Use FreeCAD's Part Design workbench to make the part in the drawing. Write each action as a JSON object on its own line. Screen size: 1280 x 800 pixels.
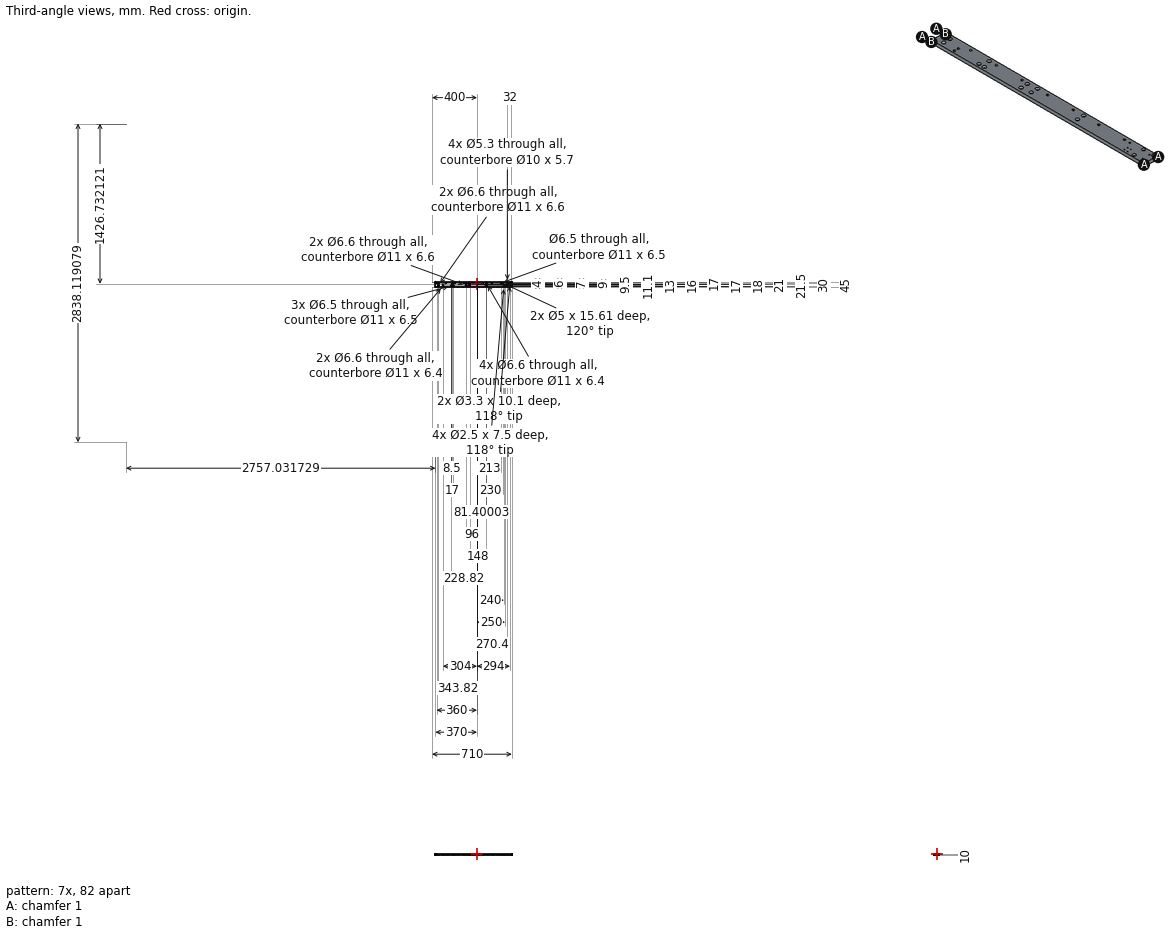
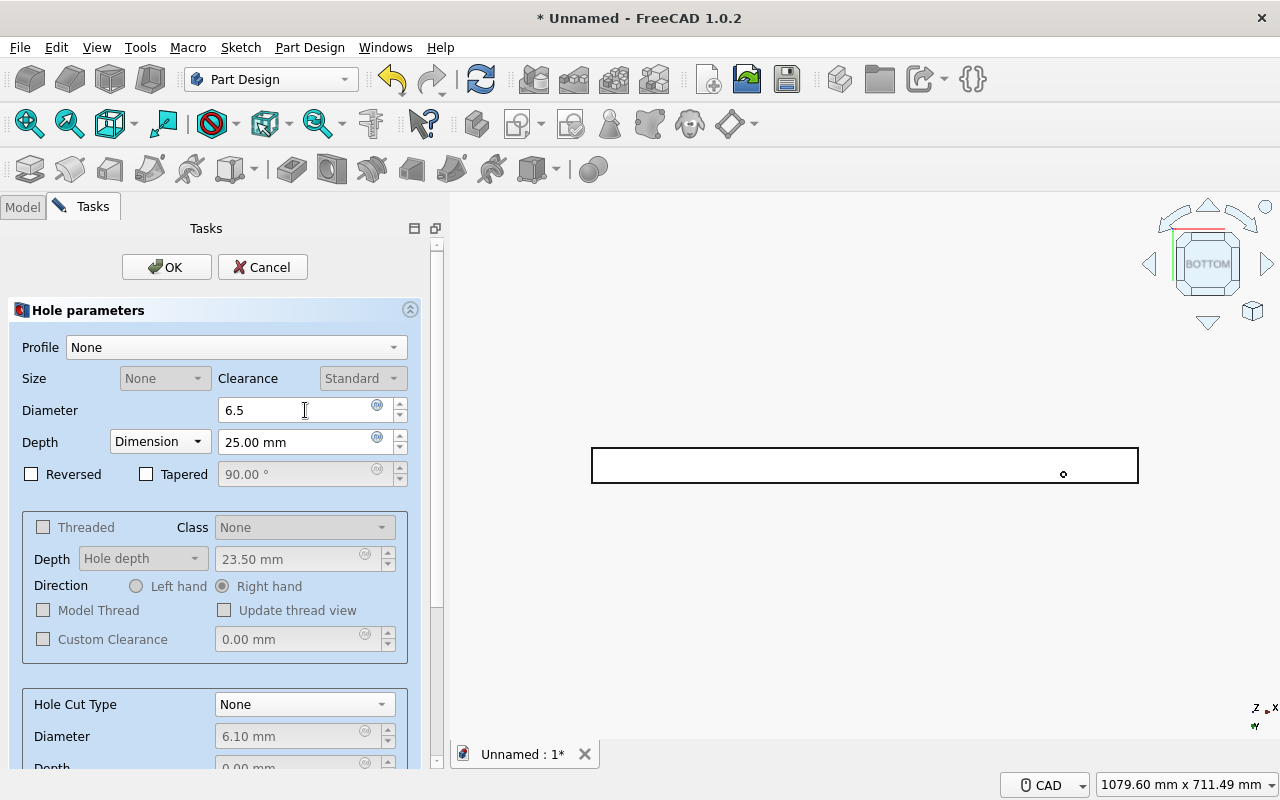
{"action": "left_click", "coordinate": [161, 442]}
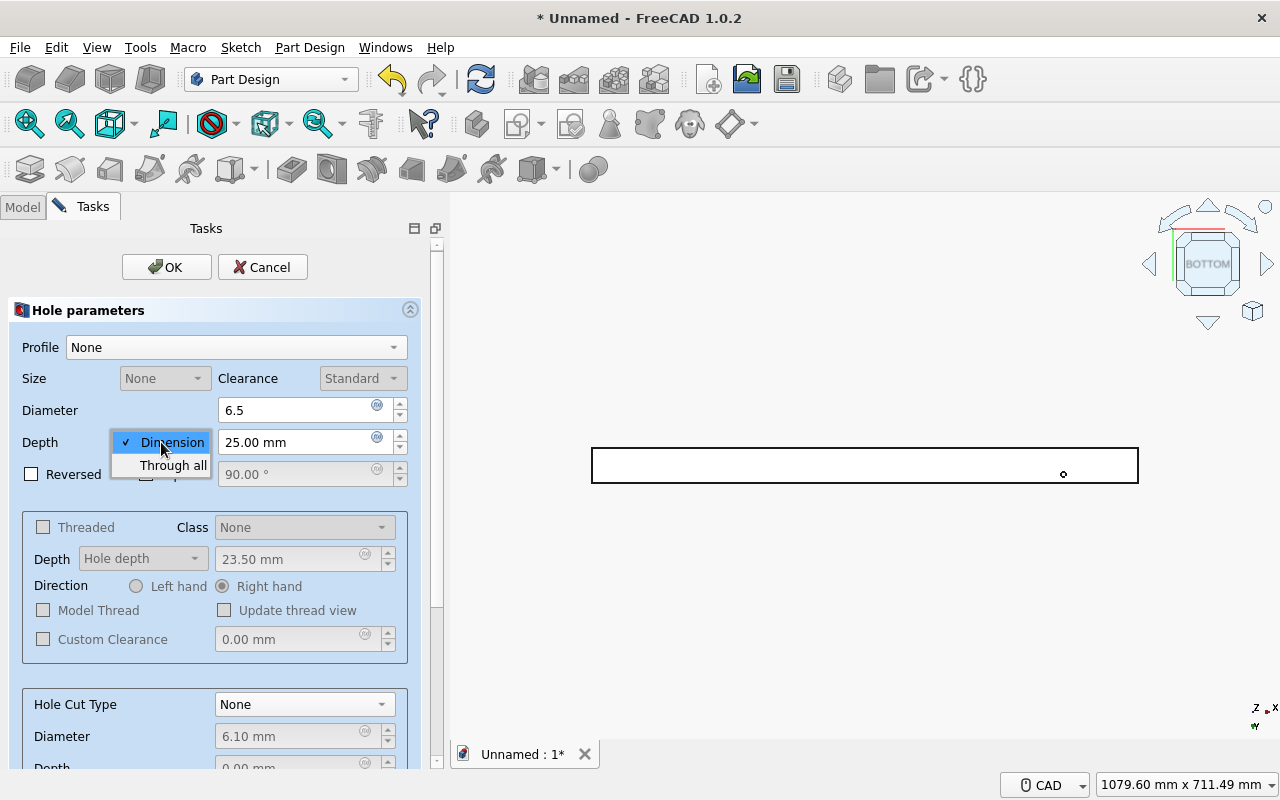
{"action": "left_click", "coordinate": [160, 466]}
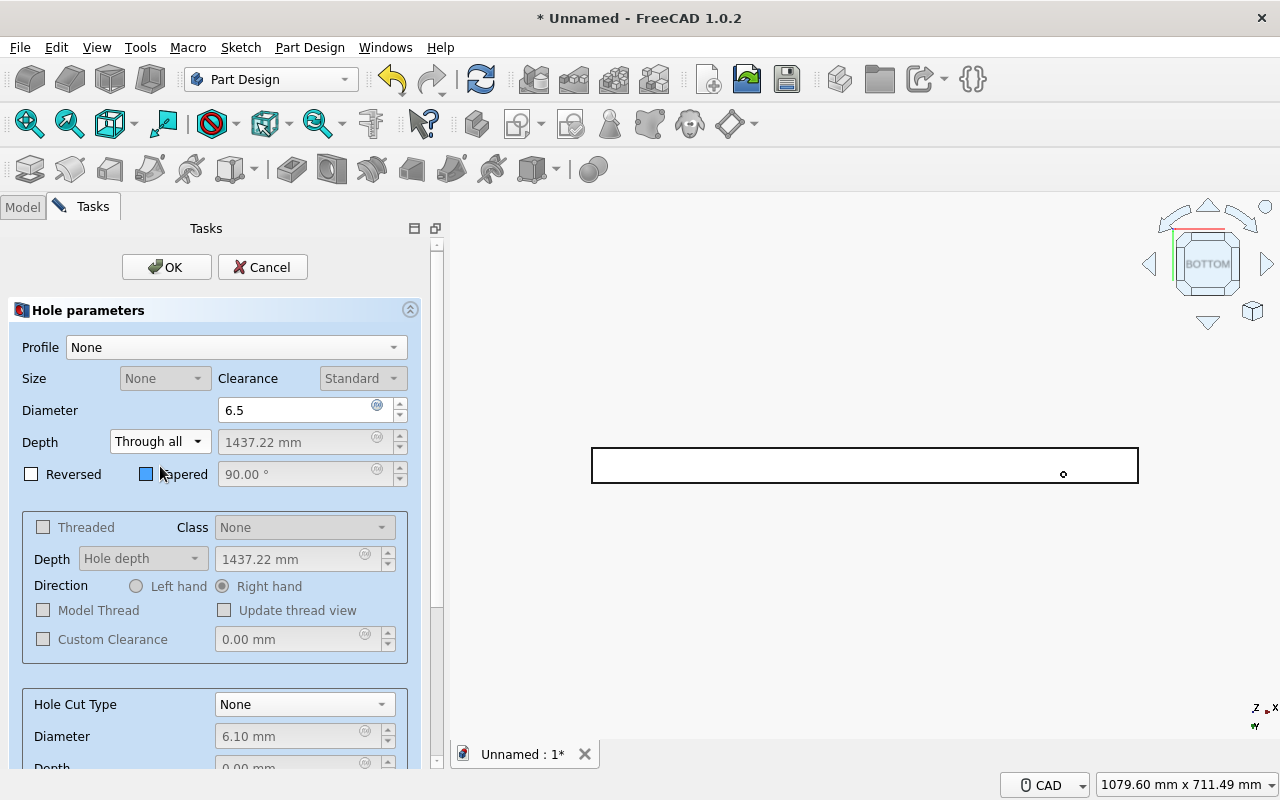
{"action": "left_click", "coordinate": [306, 704]}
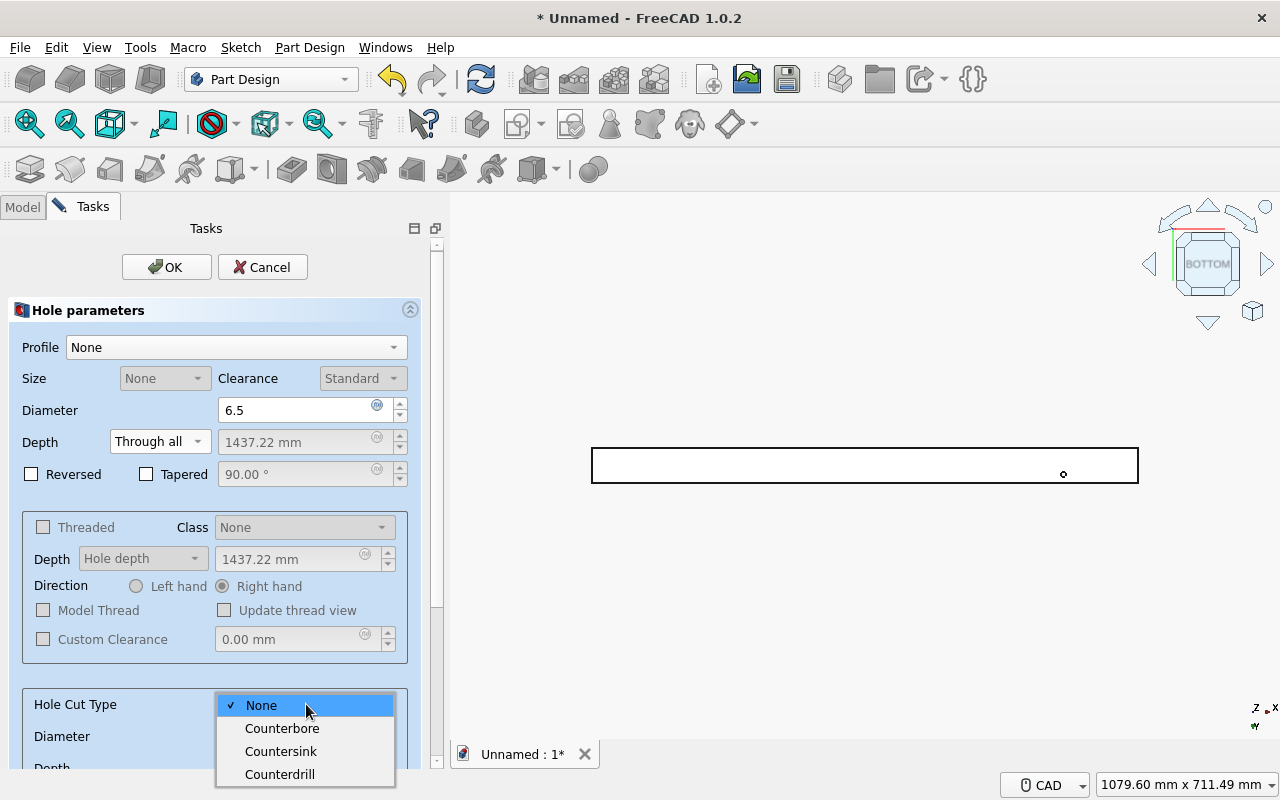
{"action": "left_click", "coordinate": [304, 728]}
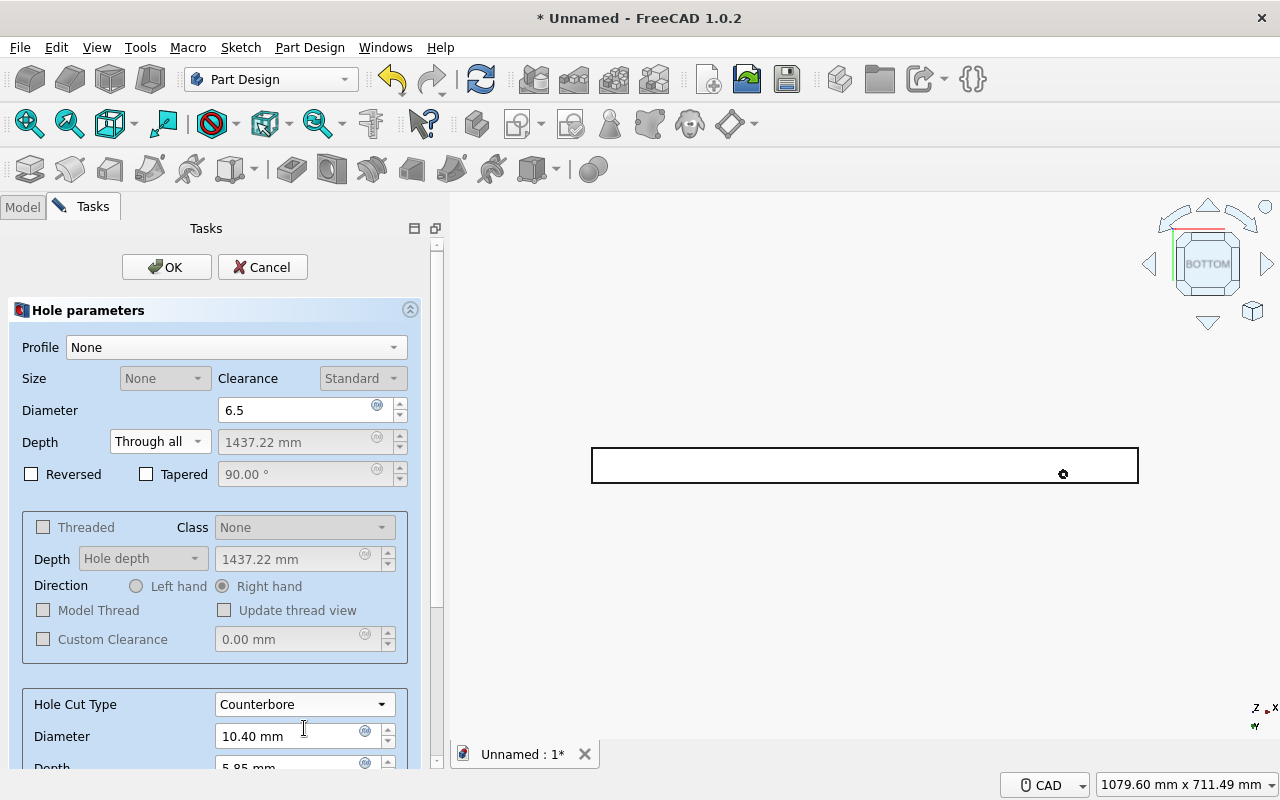
{"action": "triple_click", "coordinate": [298, 736]}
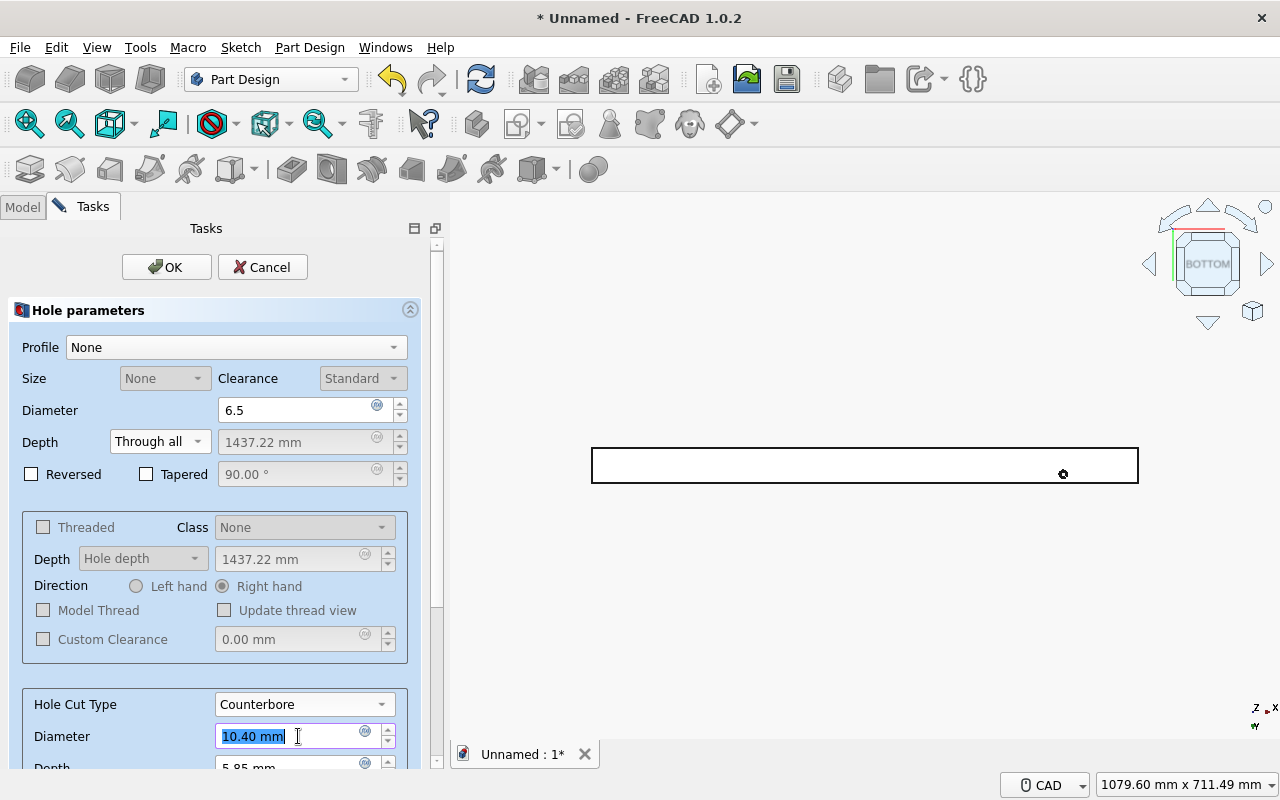
{"action": "type", "text": "11"}
{"action": "key", "text": "Tab"}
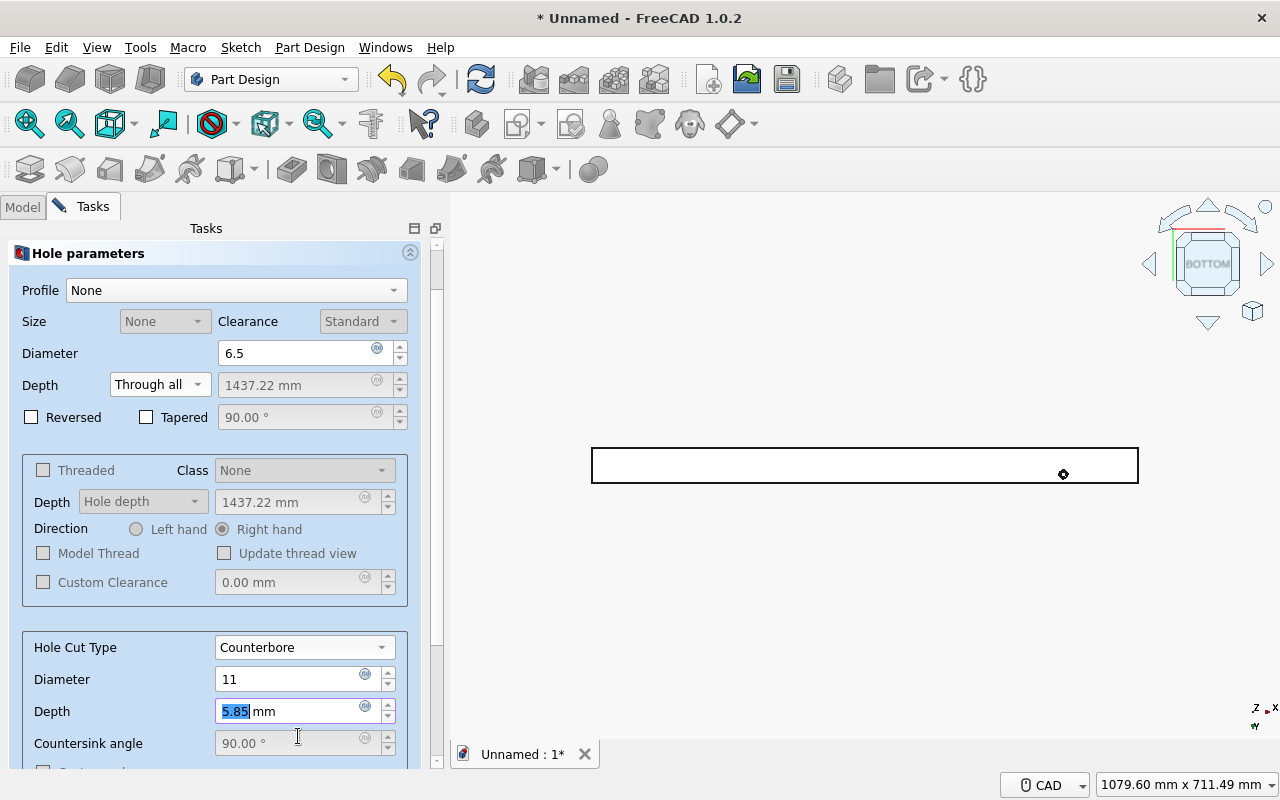
{"action": "type", "text": "6.5"}
{"action": "key", "text": "Tab"}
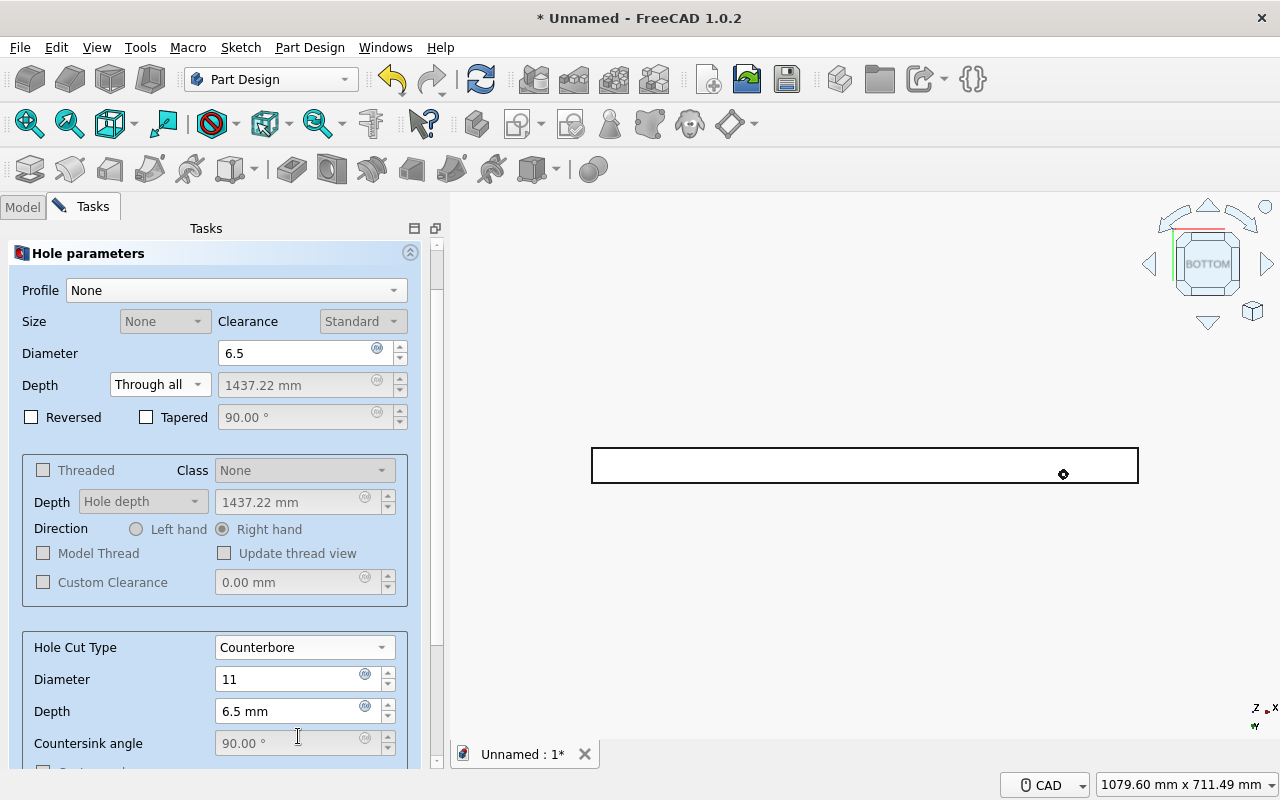
{"action": "scroll", "coordinate": [437, 503], "scroll_direction": "up", "scroll_amount": 2}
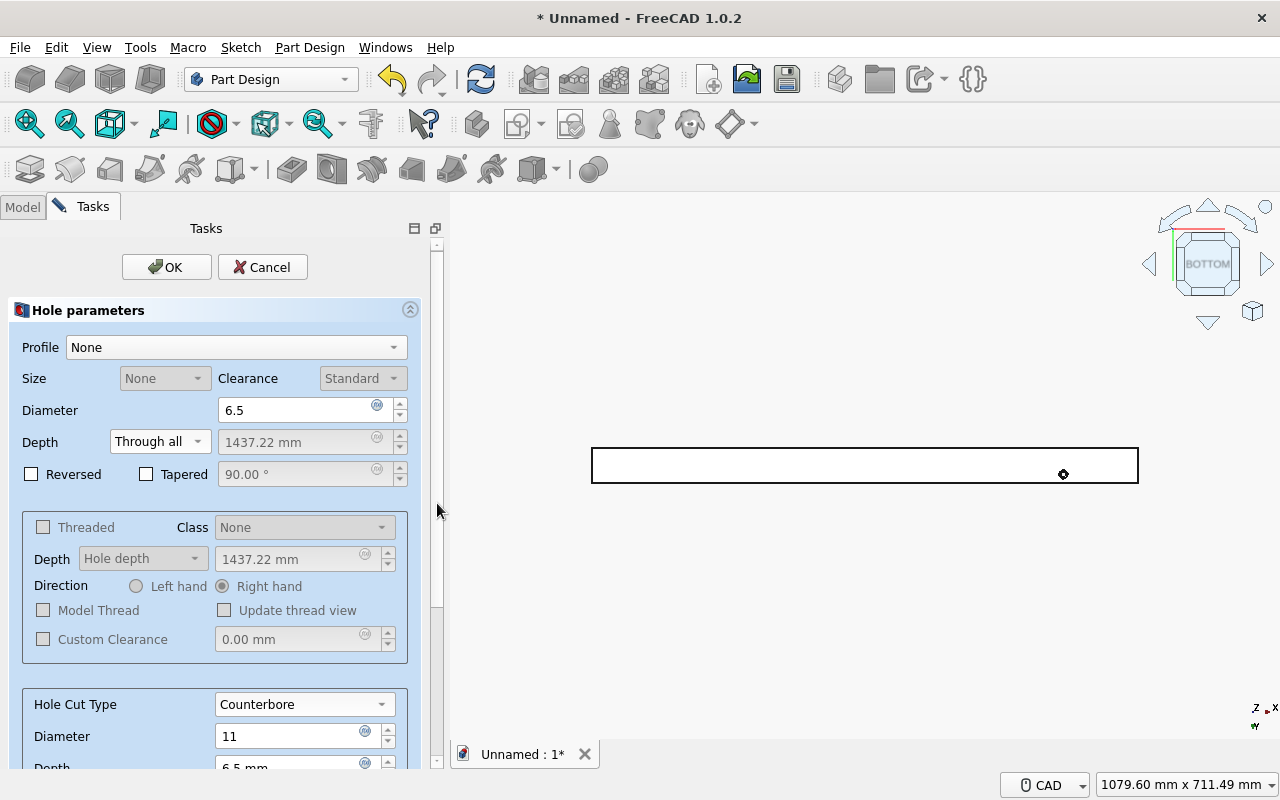
{"action": "left_click", "coordinate": [167, 267]}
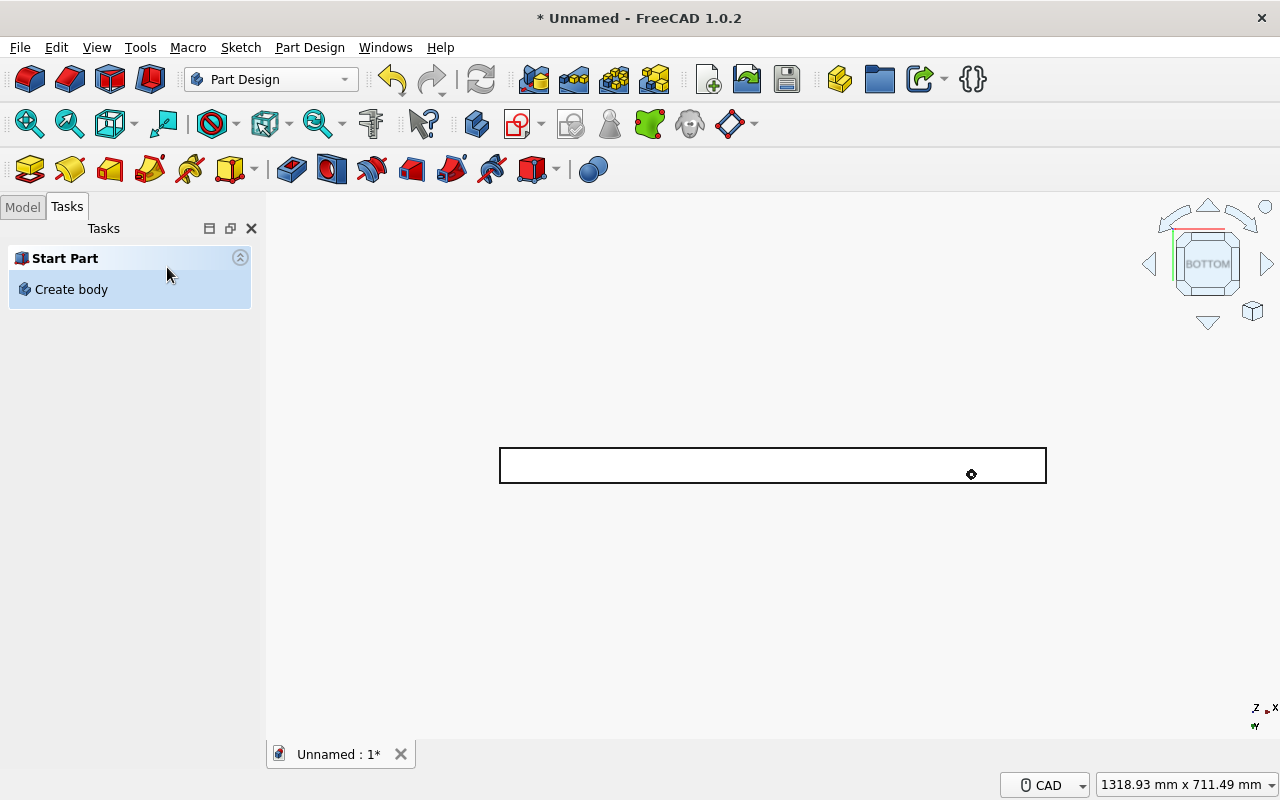
{"action": "left_click", "coordinate": [23, 206]}